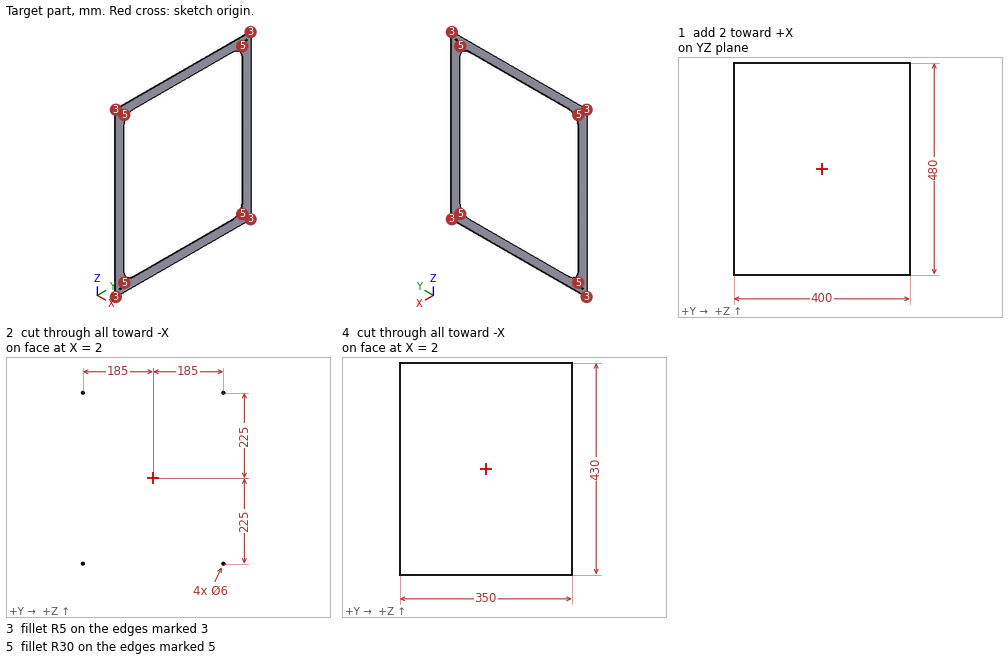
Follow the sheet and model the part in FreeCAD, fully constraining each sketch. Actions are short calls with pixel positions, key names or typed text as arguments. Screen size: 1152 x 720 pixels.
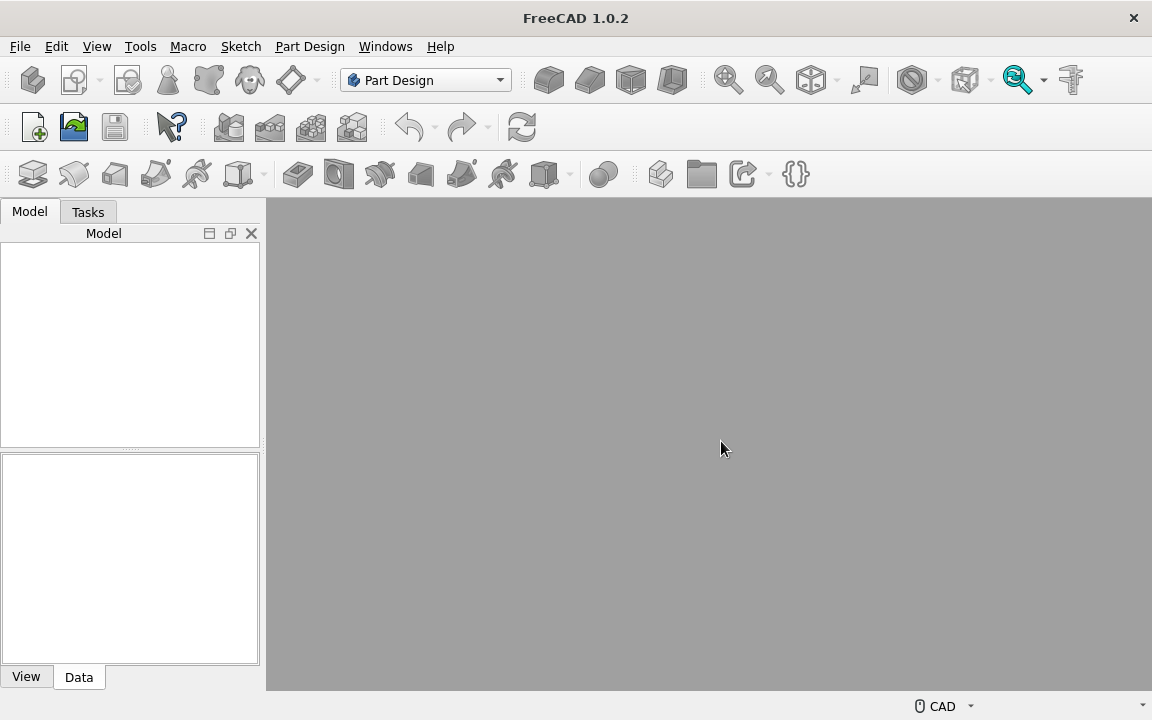
click(33, 128)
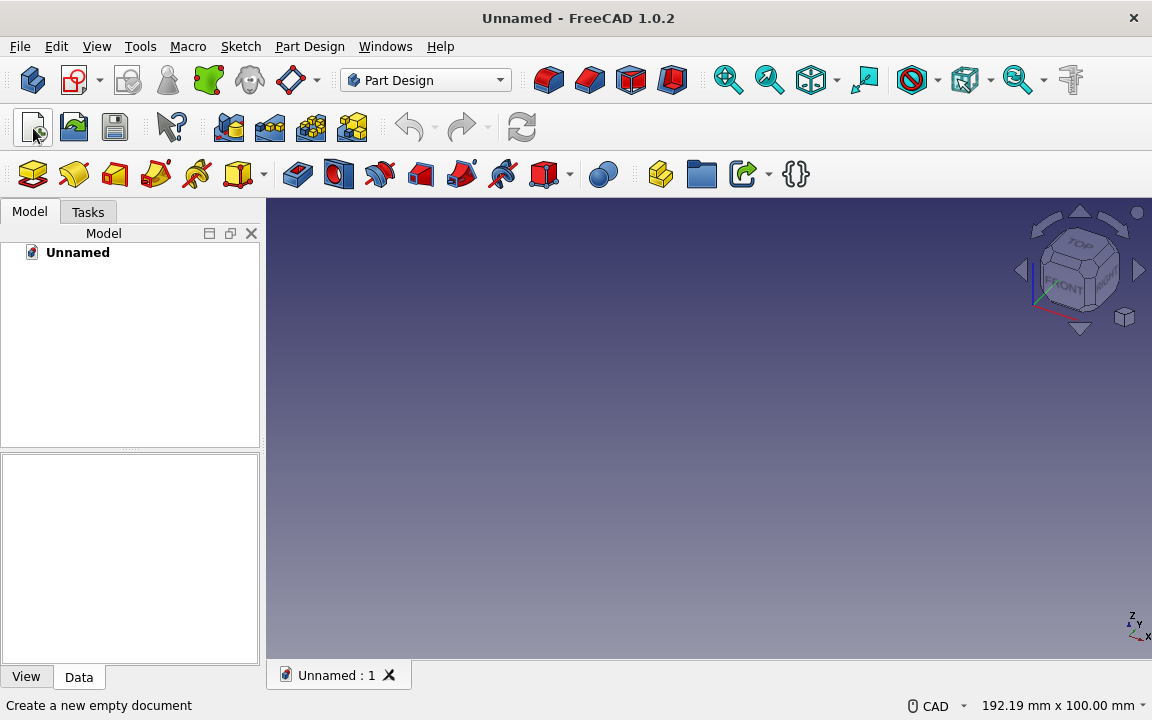
click(74, 80)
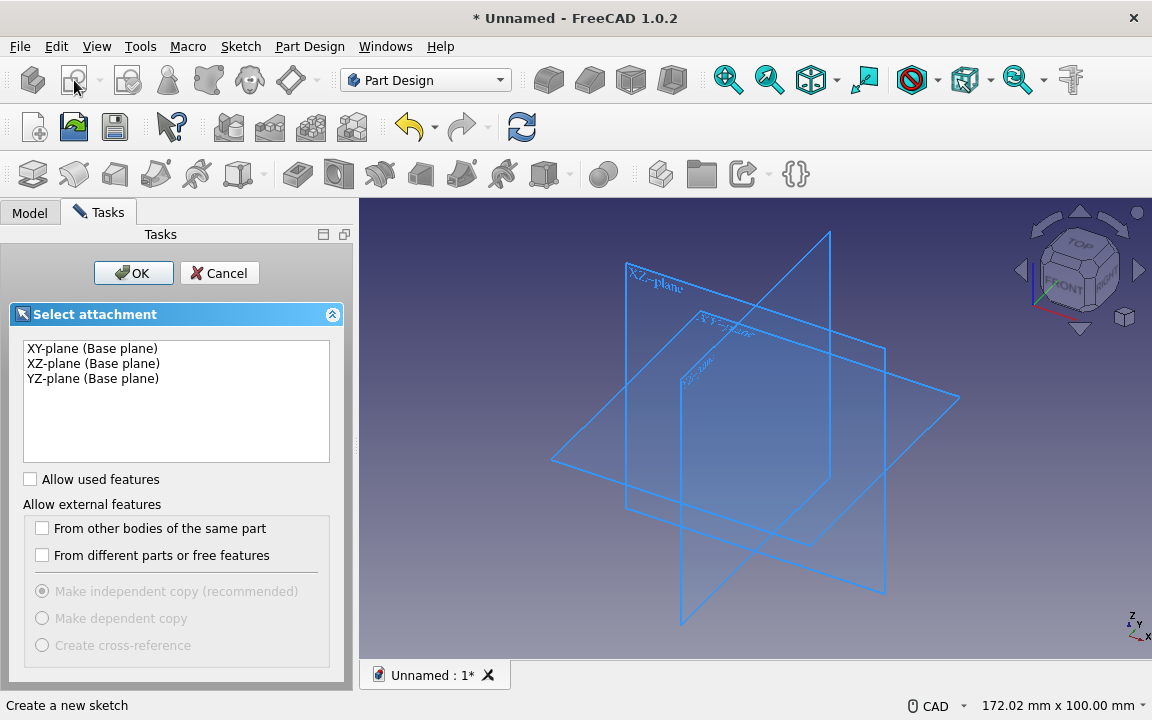
click(84, 378)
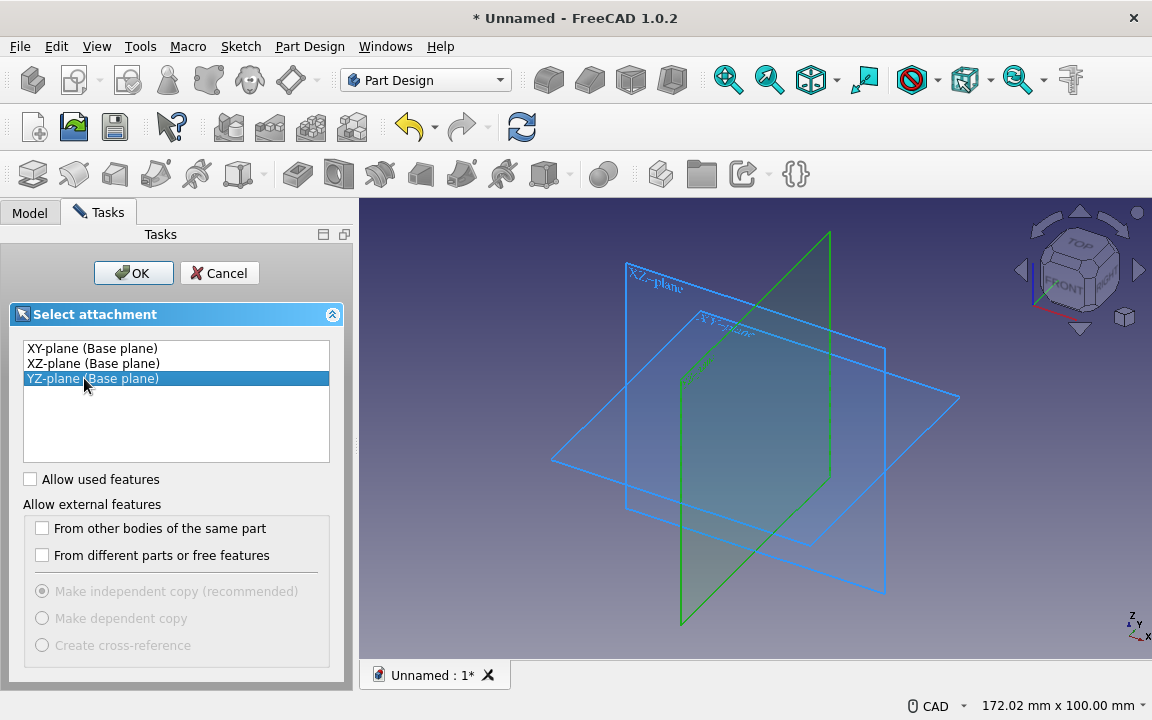
click(134, 273)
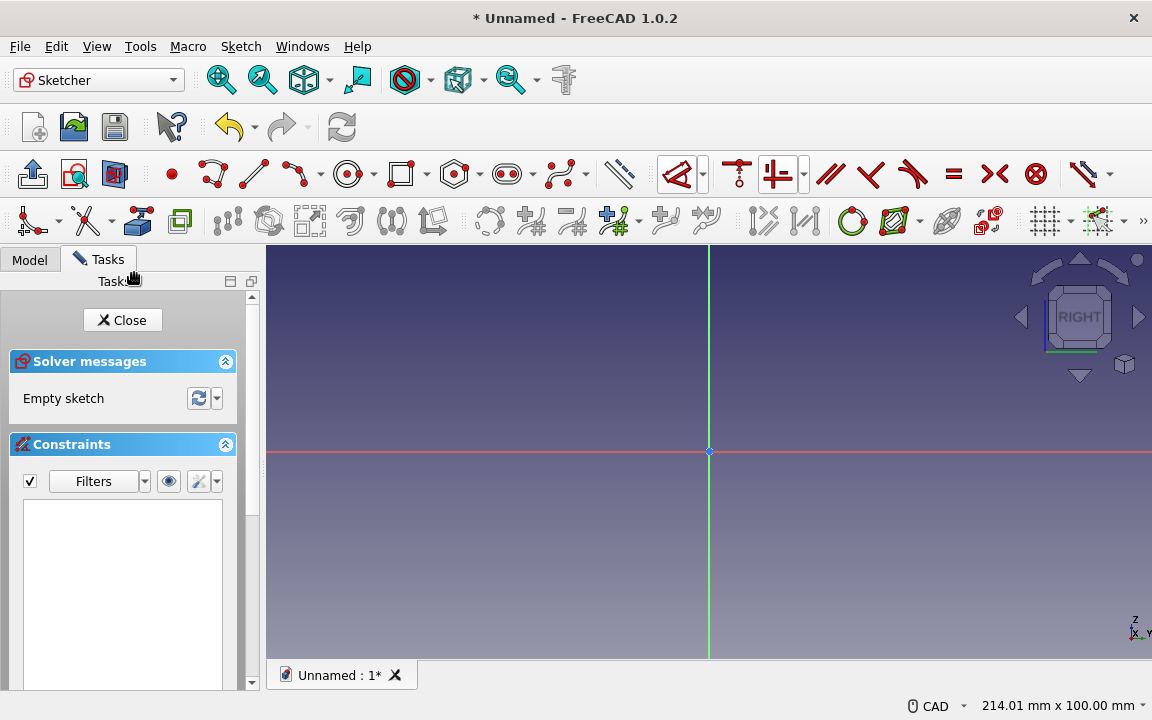
scroll(630, 452, down, 10)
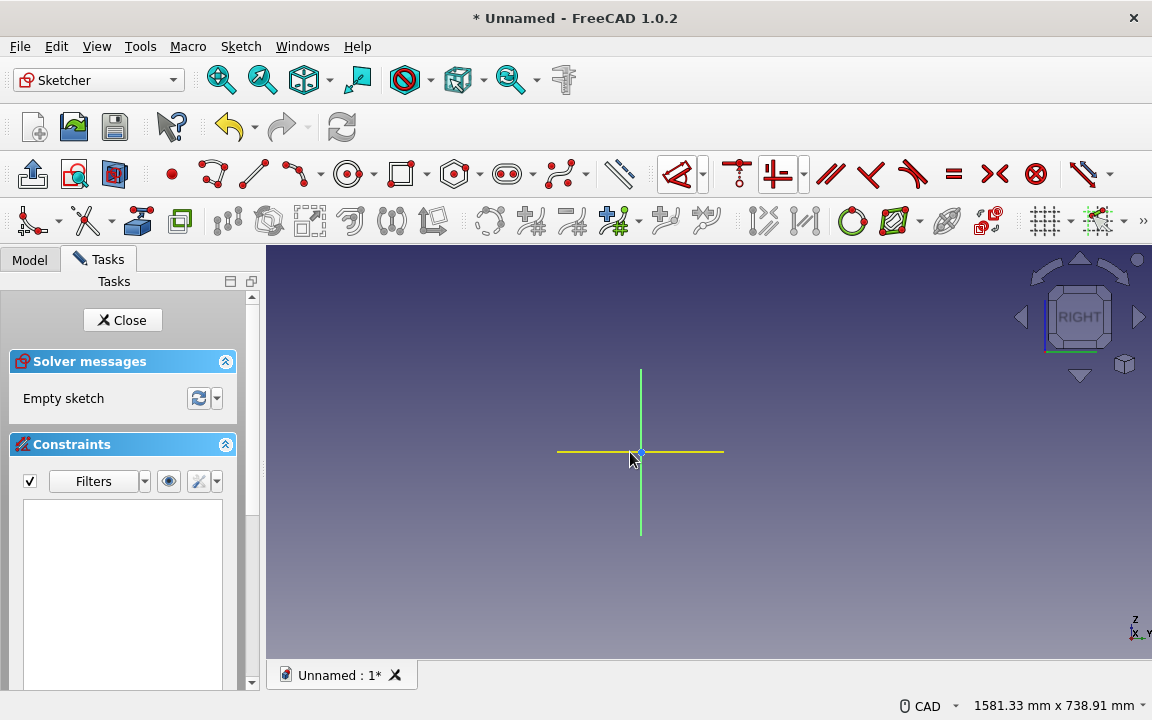
key(g)
key(v)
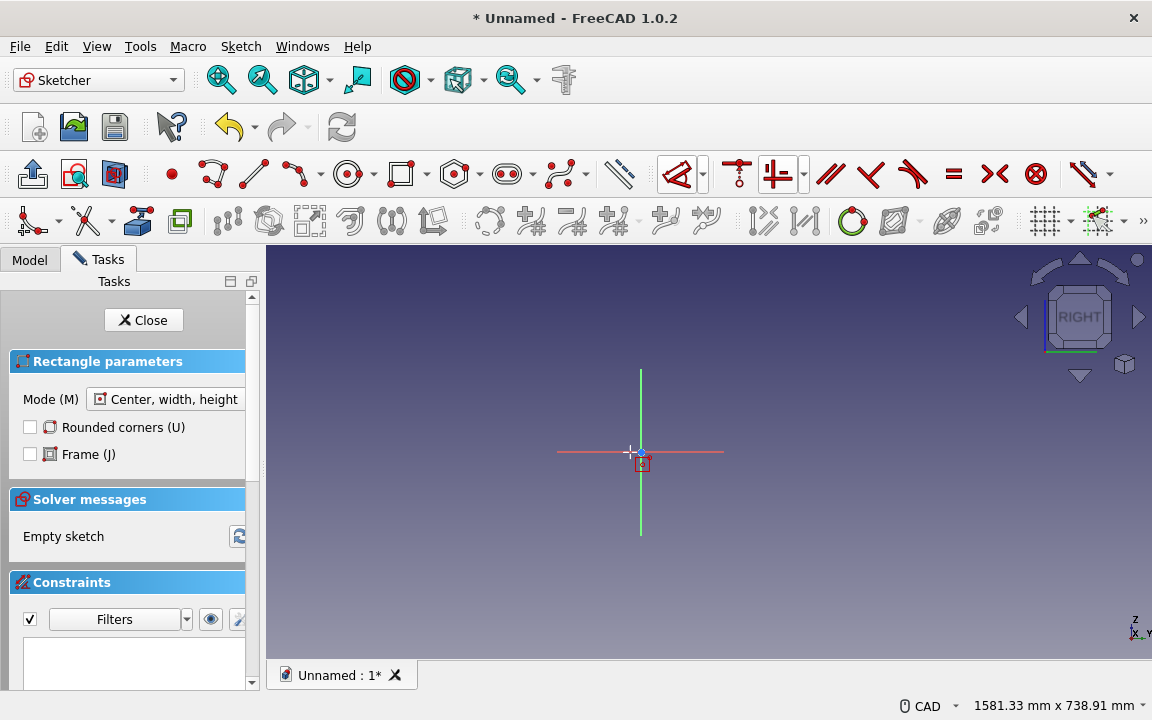
click(641, 452)
move(753, 318)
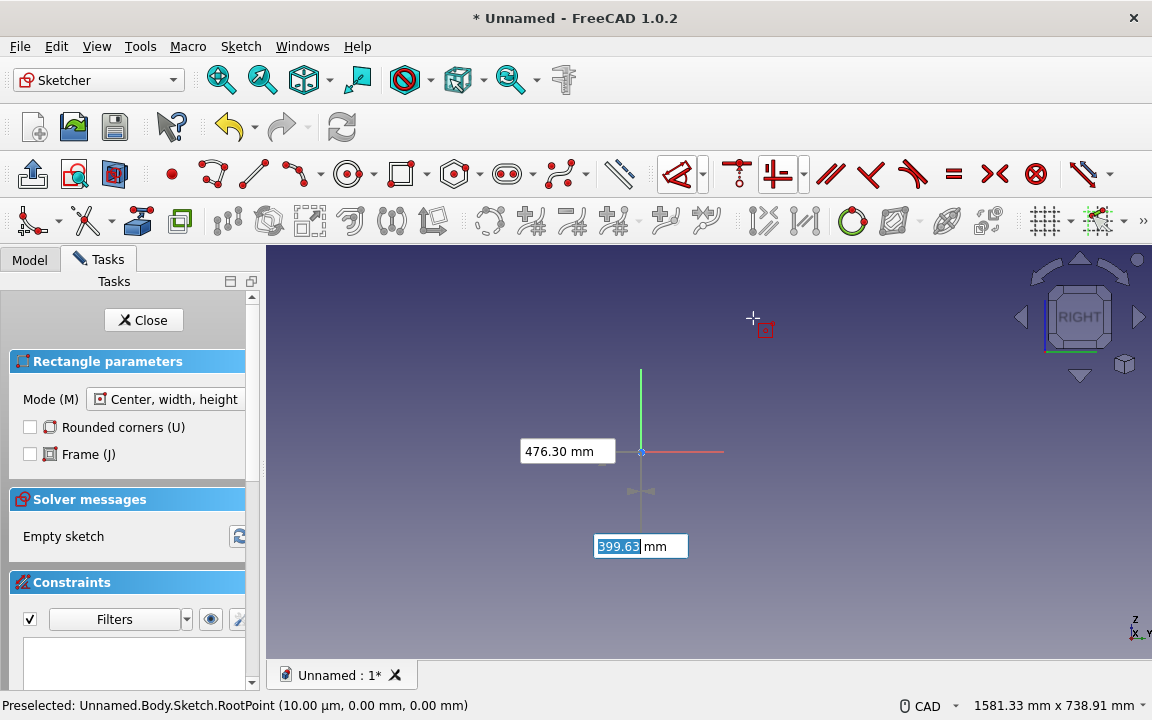
text(400)
key(Tab)
text(480)
key(Return)
key(Escape)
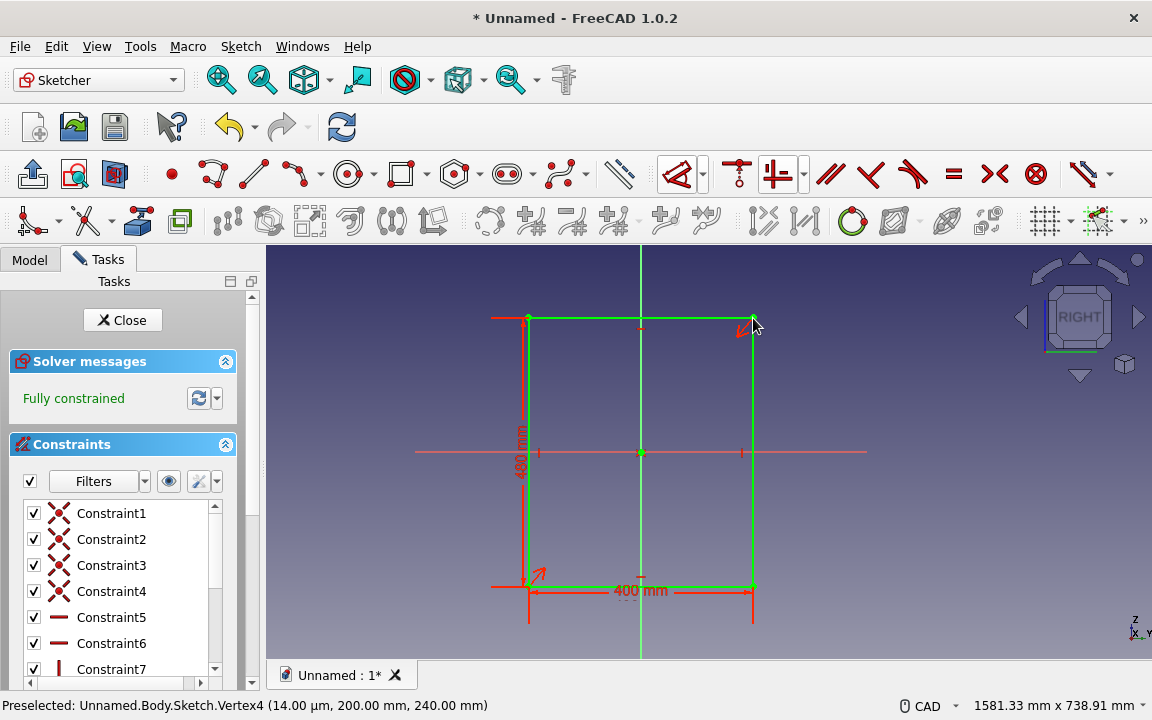
click(123, 320)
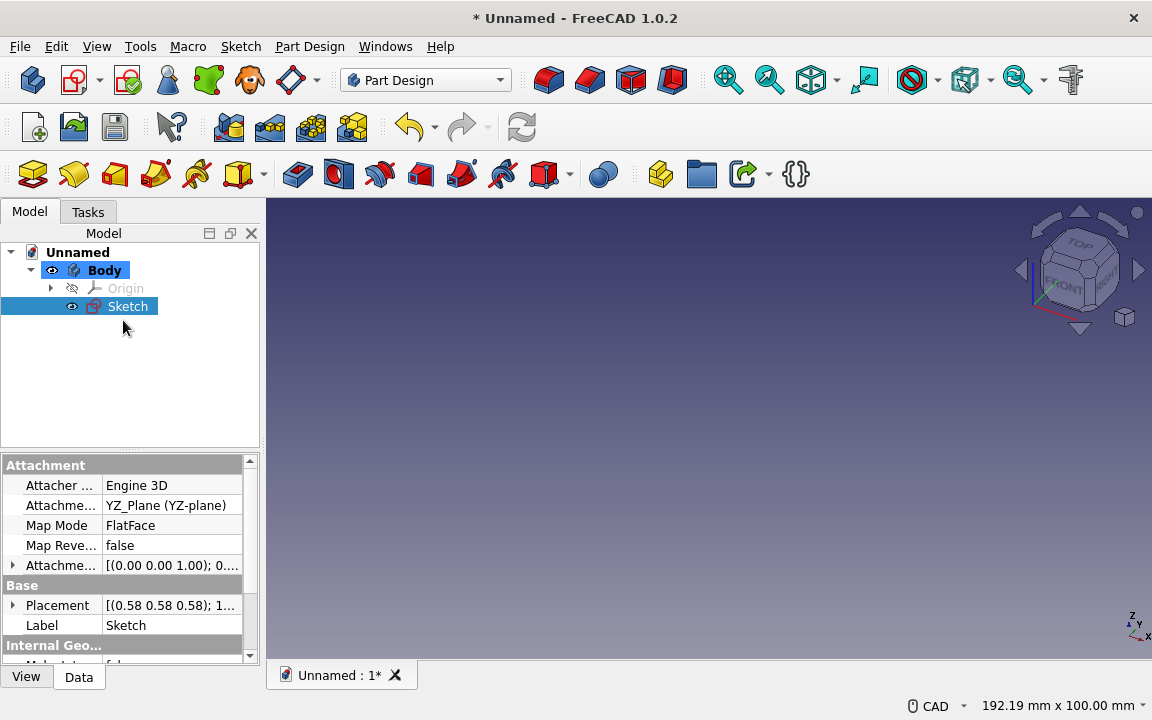
click(33, 174)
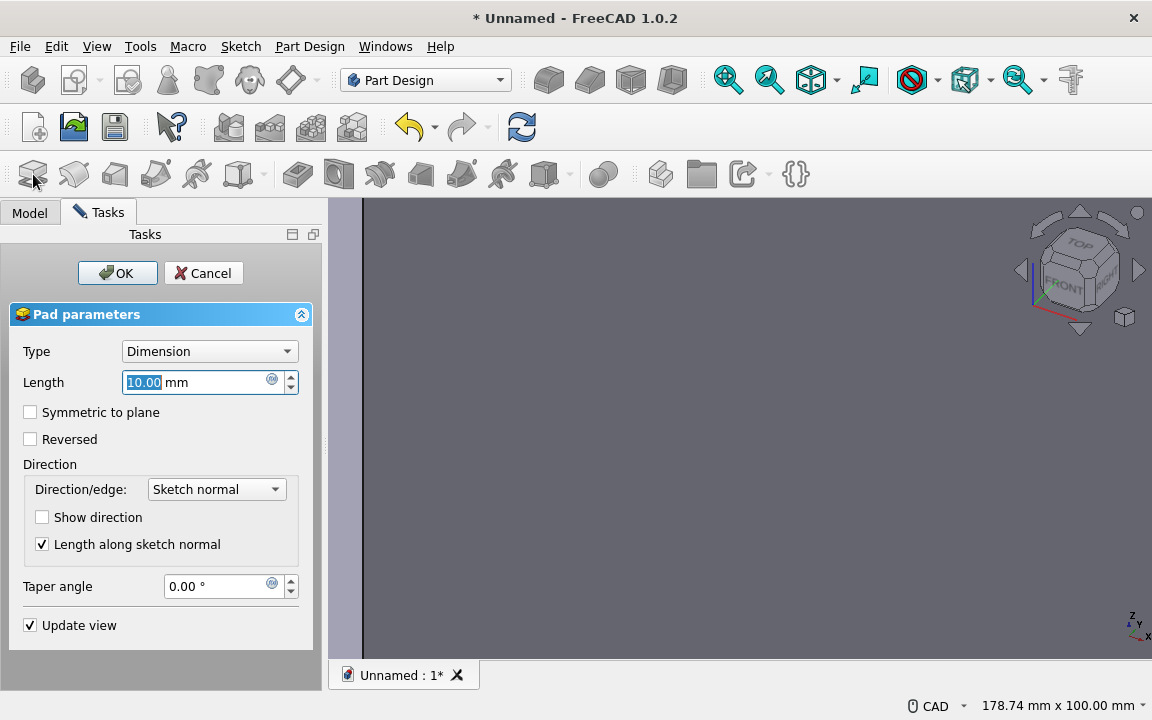
text(2)
key(Tab)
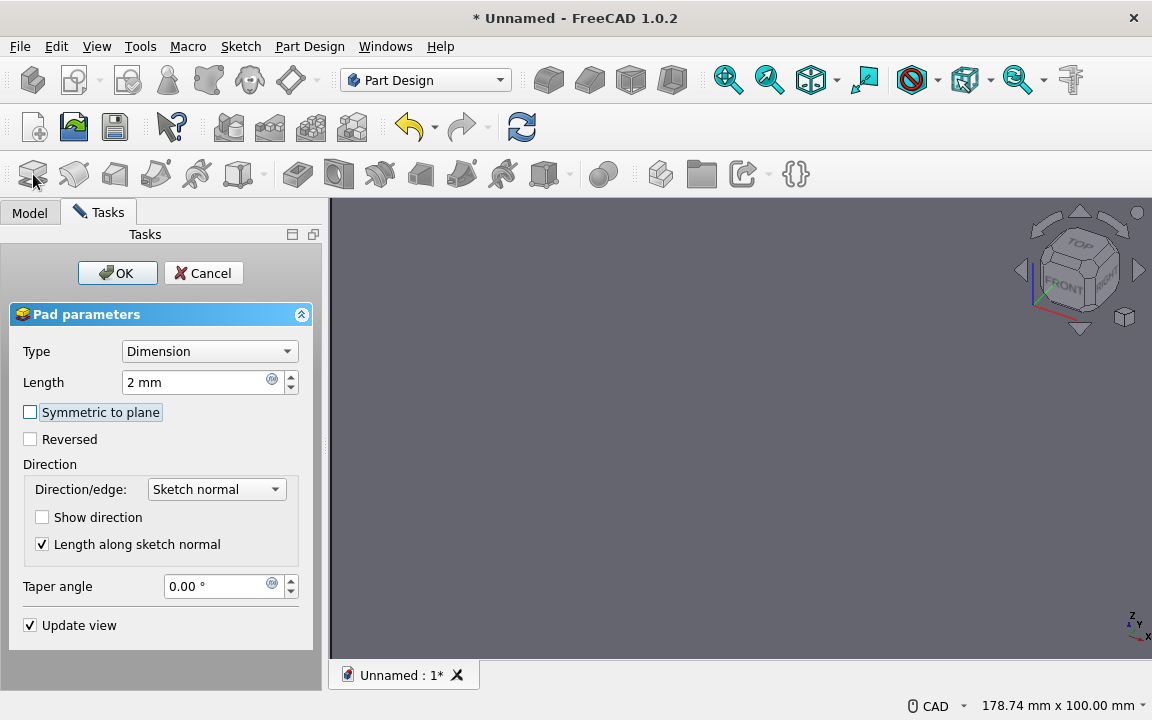
click(118, 273)